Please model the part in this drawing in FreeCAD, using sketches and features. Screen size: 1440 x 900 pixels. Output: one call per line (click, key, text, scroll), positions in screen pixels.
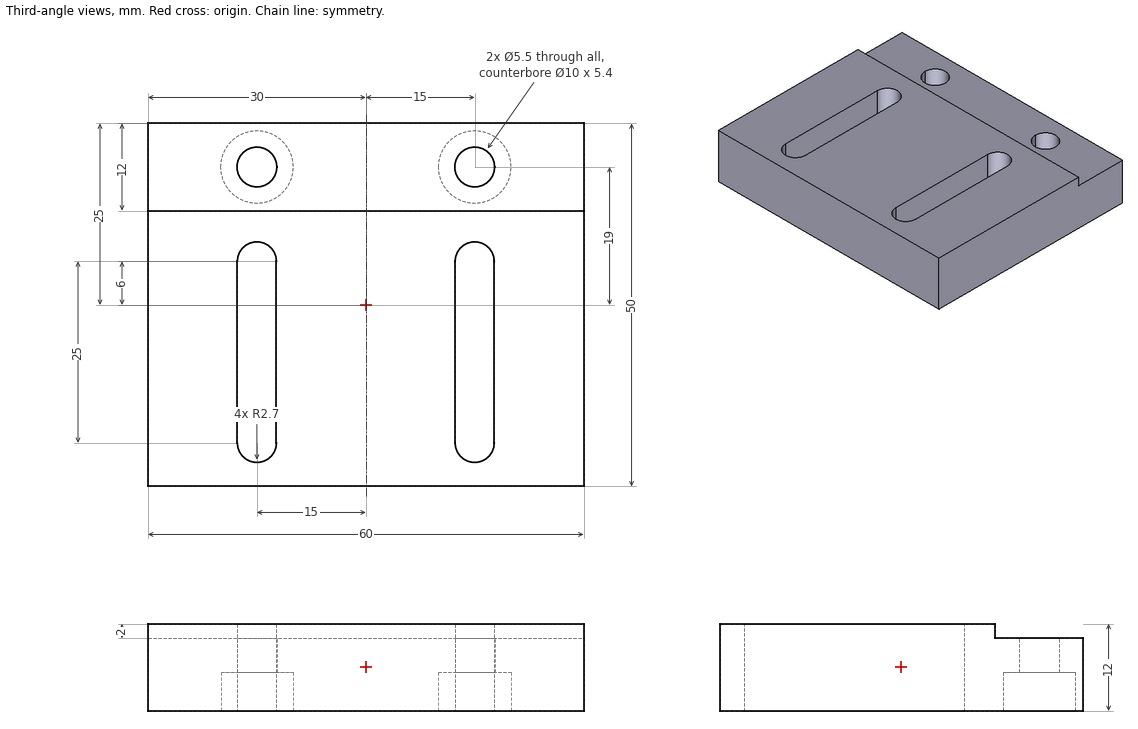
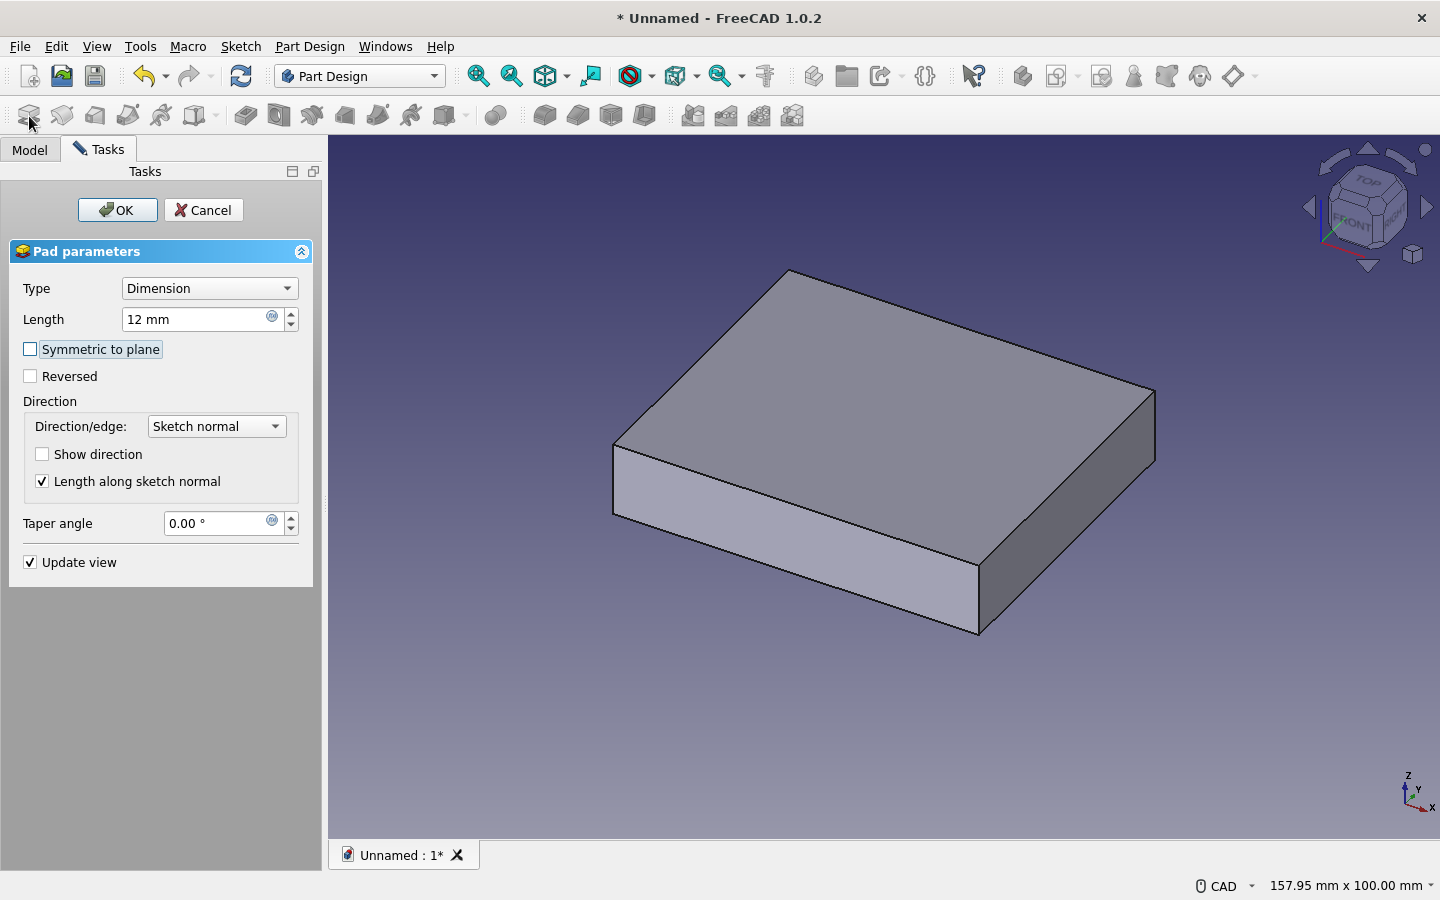
click(31, 349)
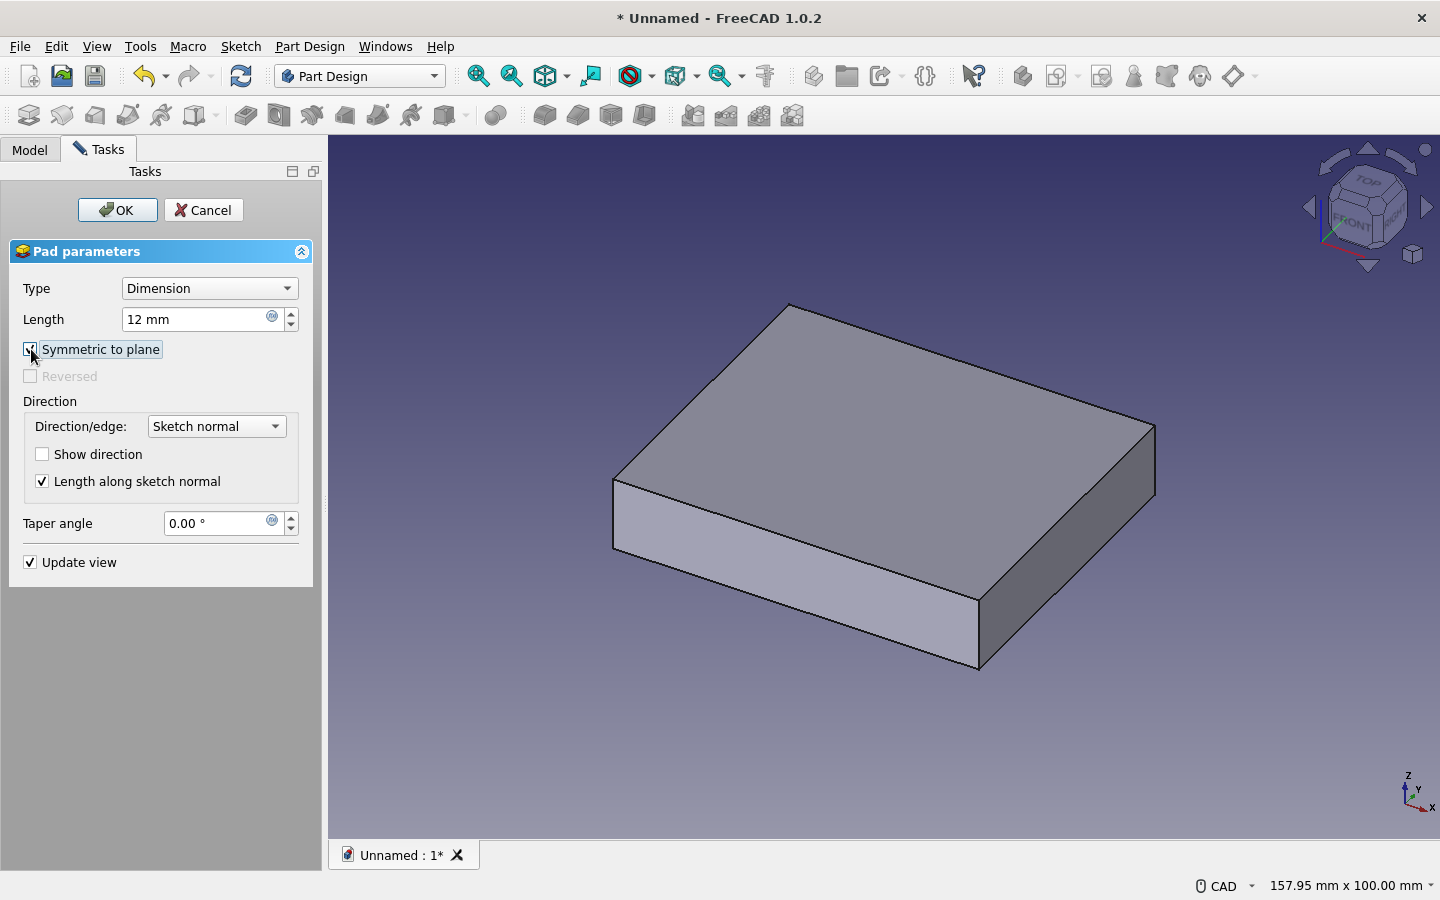
click(118, 210)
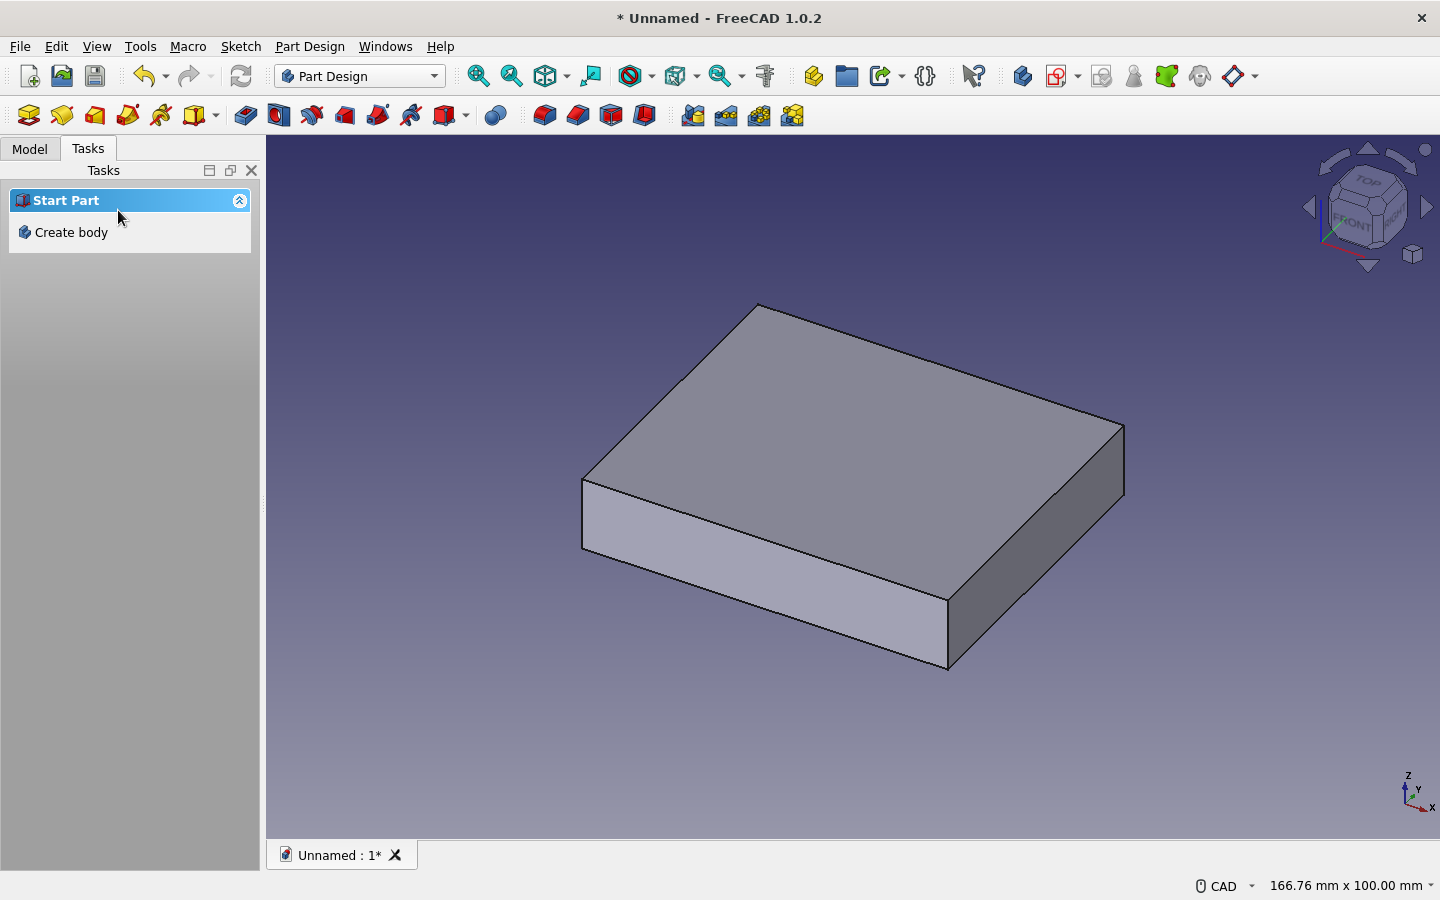
click(853, 451)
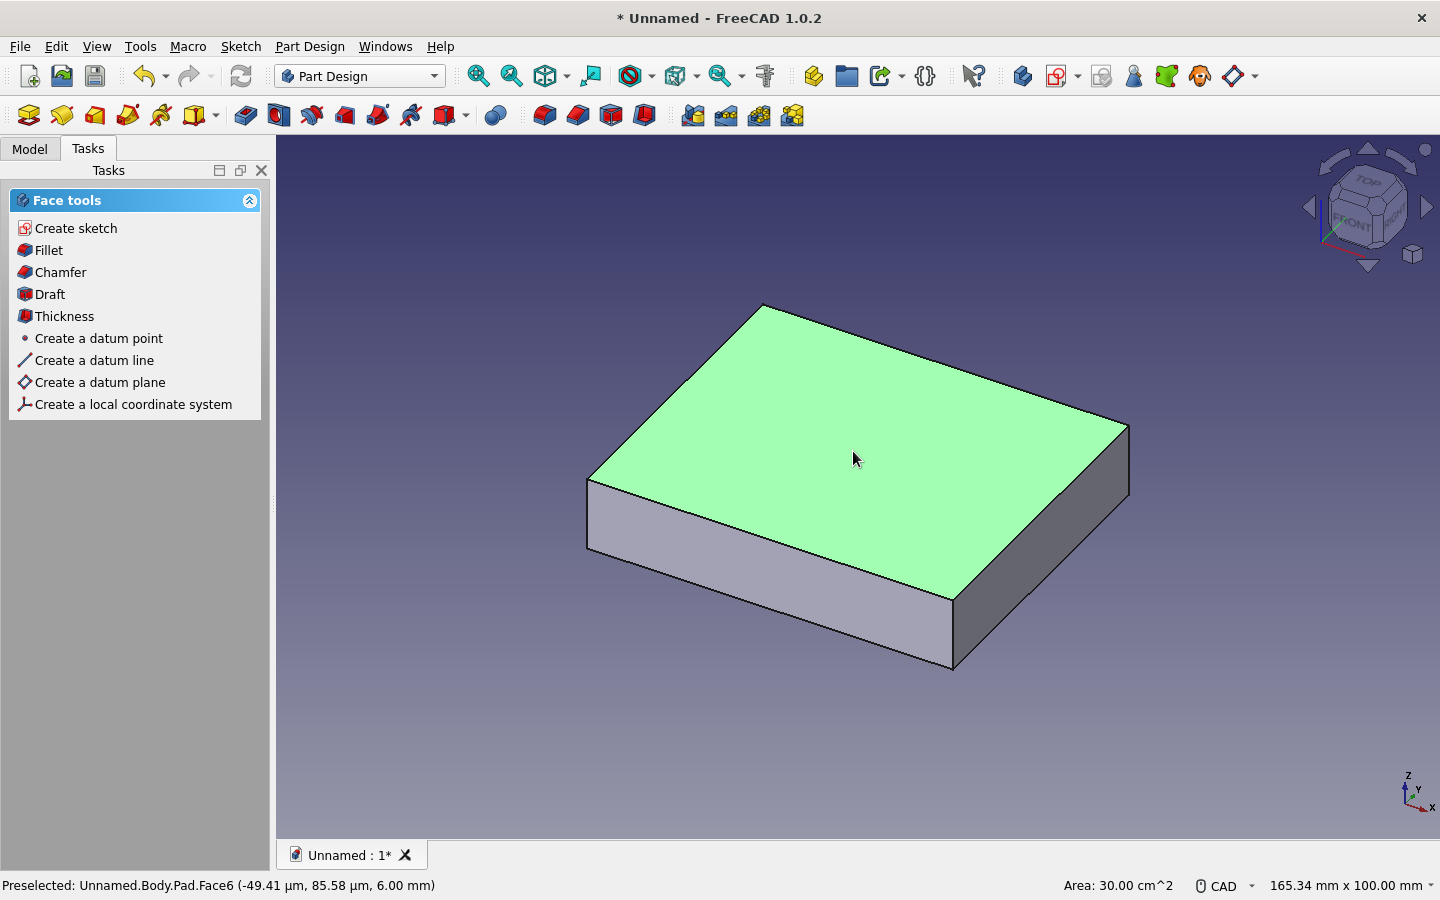
click(1056, 76)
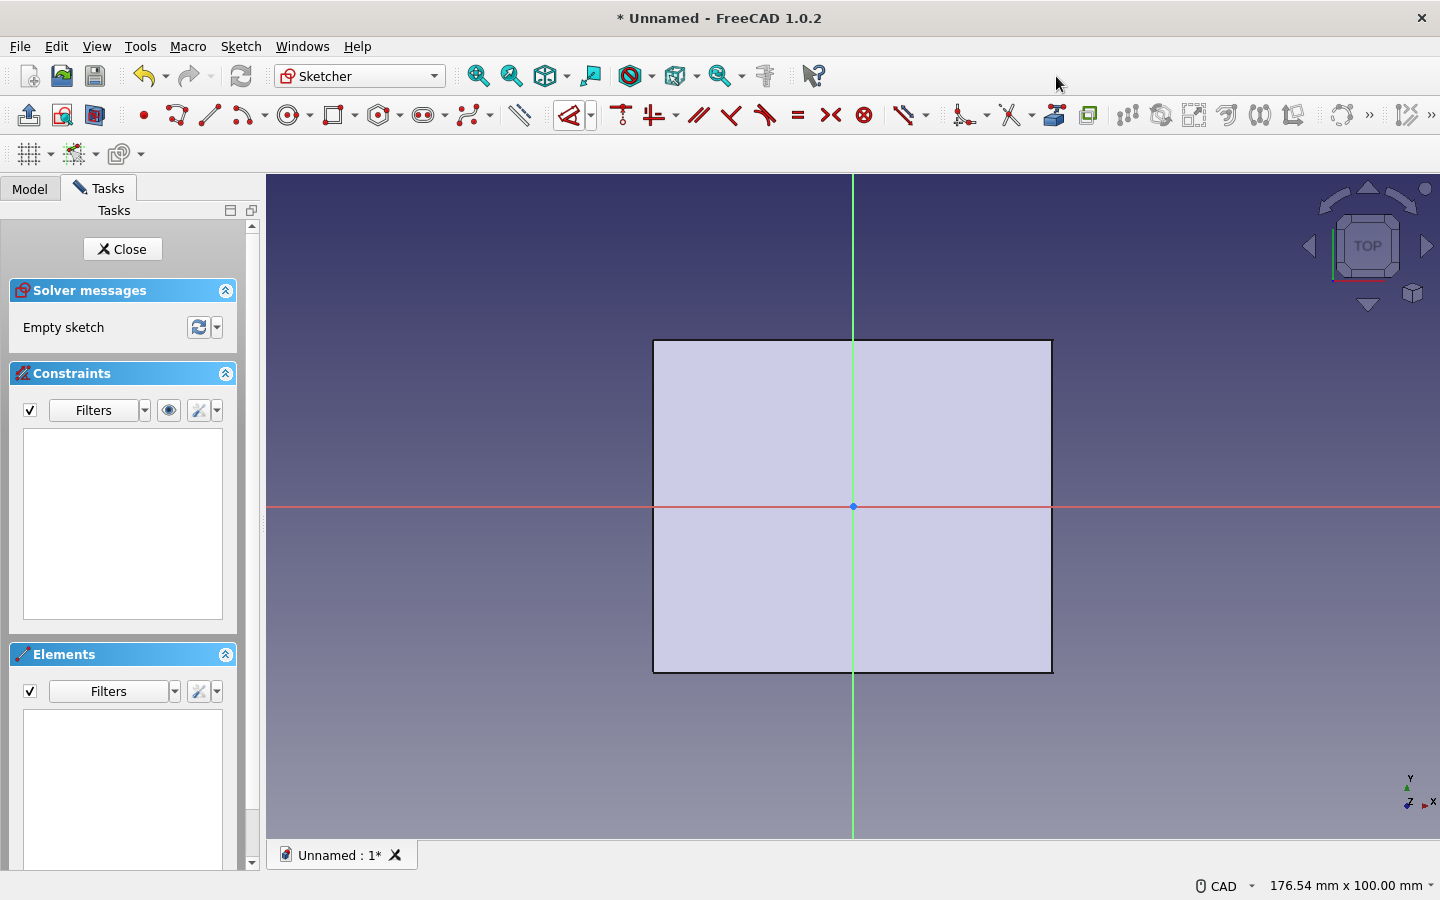
scroll(936, 322, up, 3)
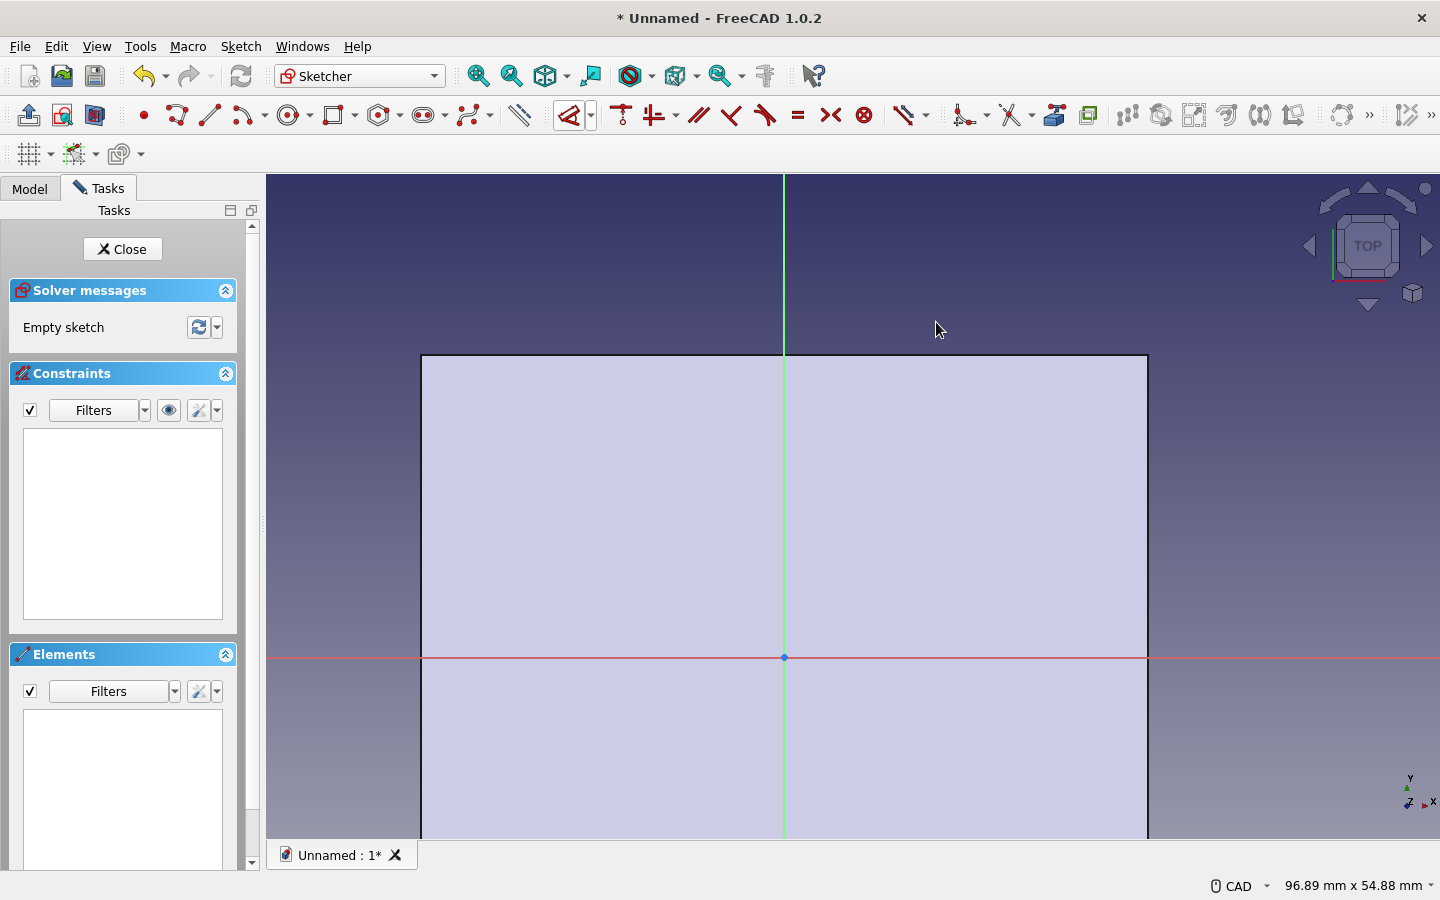
click(332, 116)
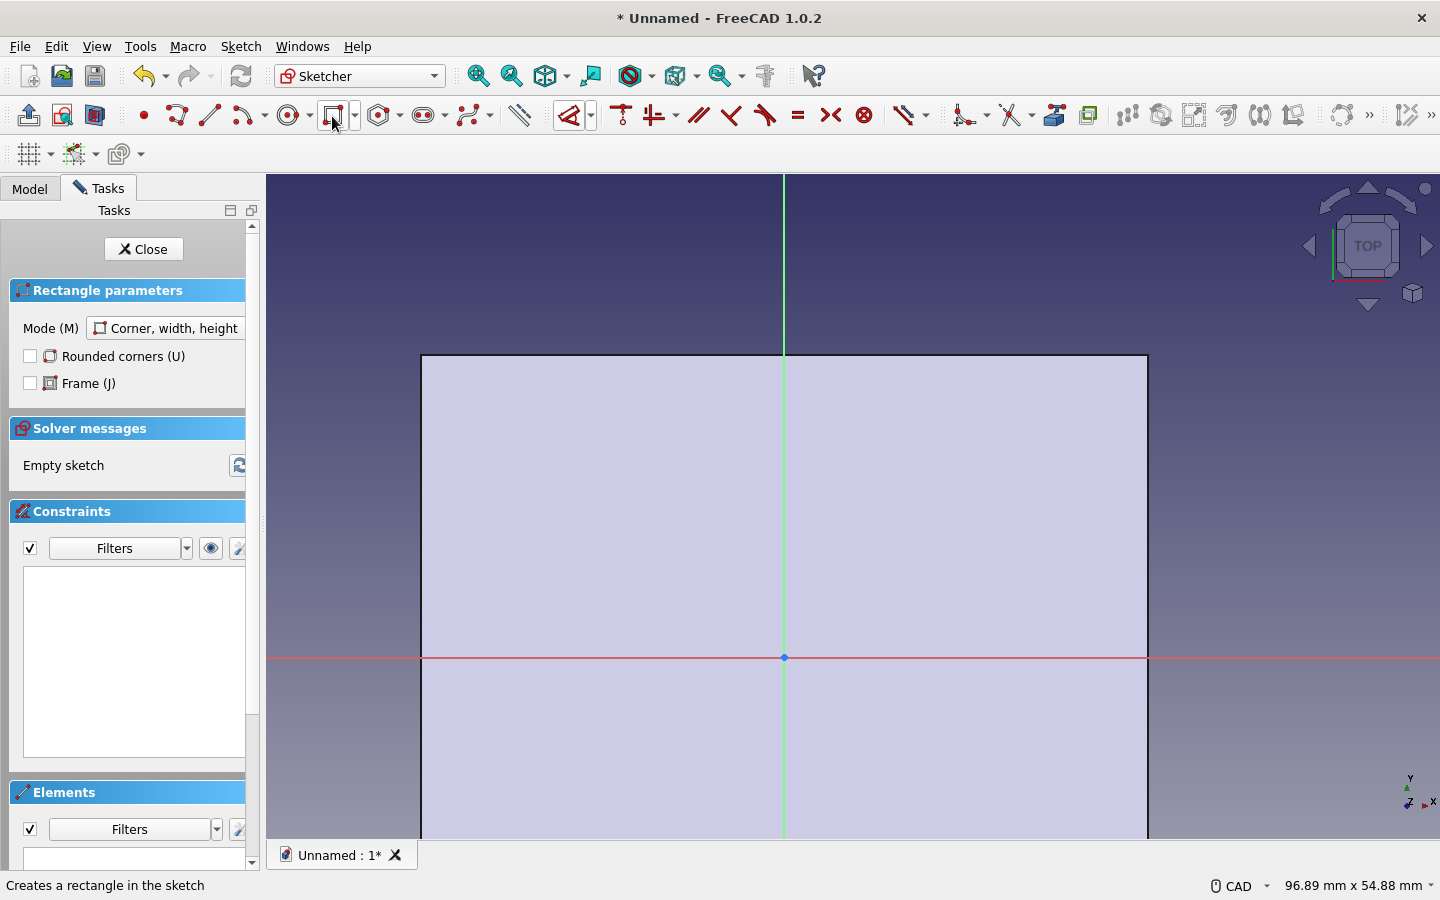
click(421, 355)
click(1148, 500)
key(Escape)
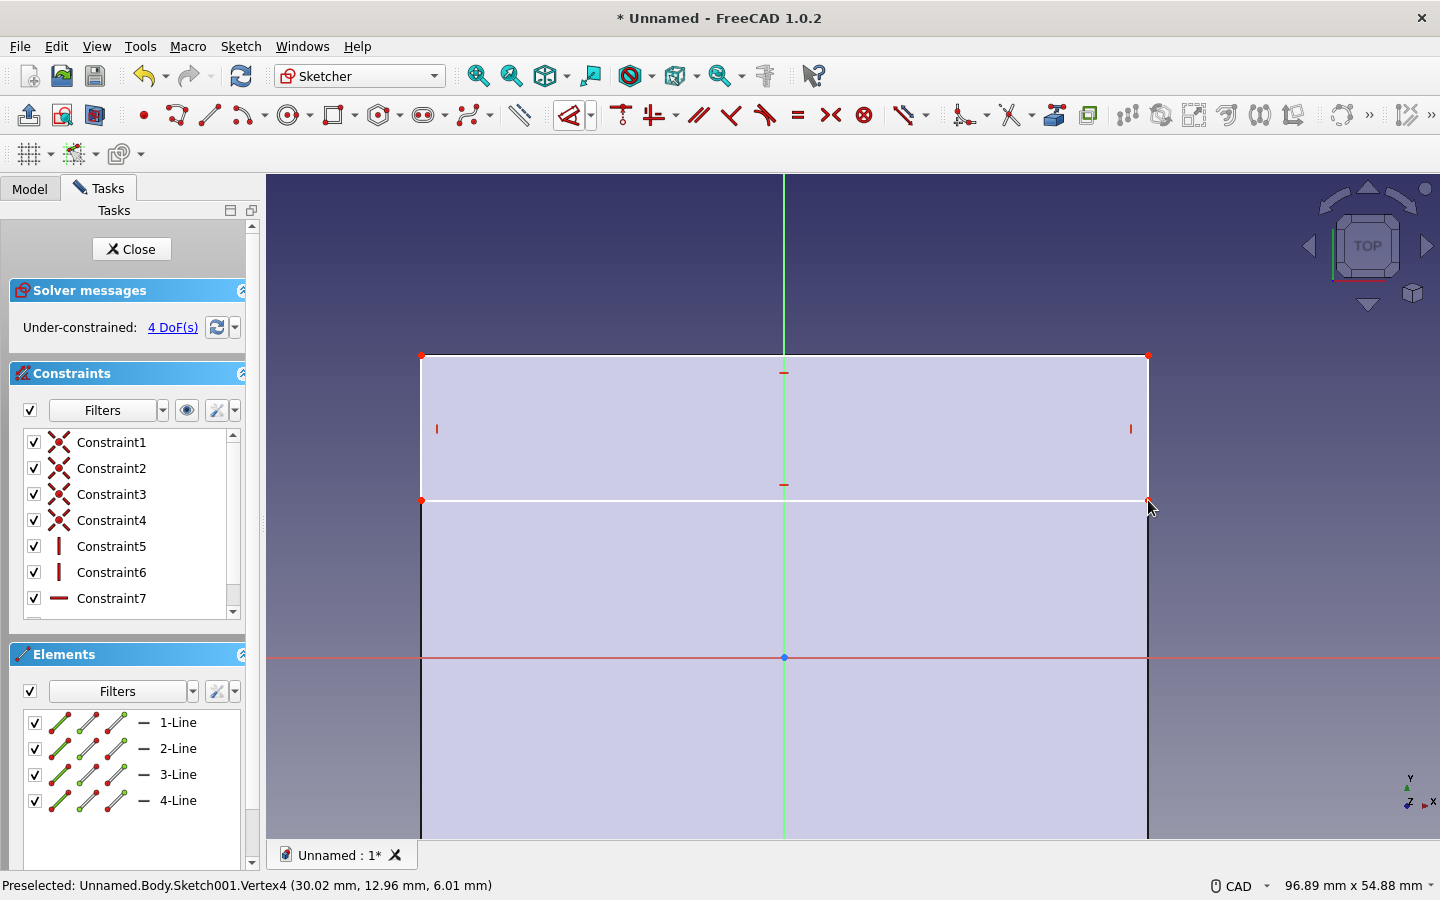
click(421, 399)